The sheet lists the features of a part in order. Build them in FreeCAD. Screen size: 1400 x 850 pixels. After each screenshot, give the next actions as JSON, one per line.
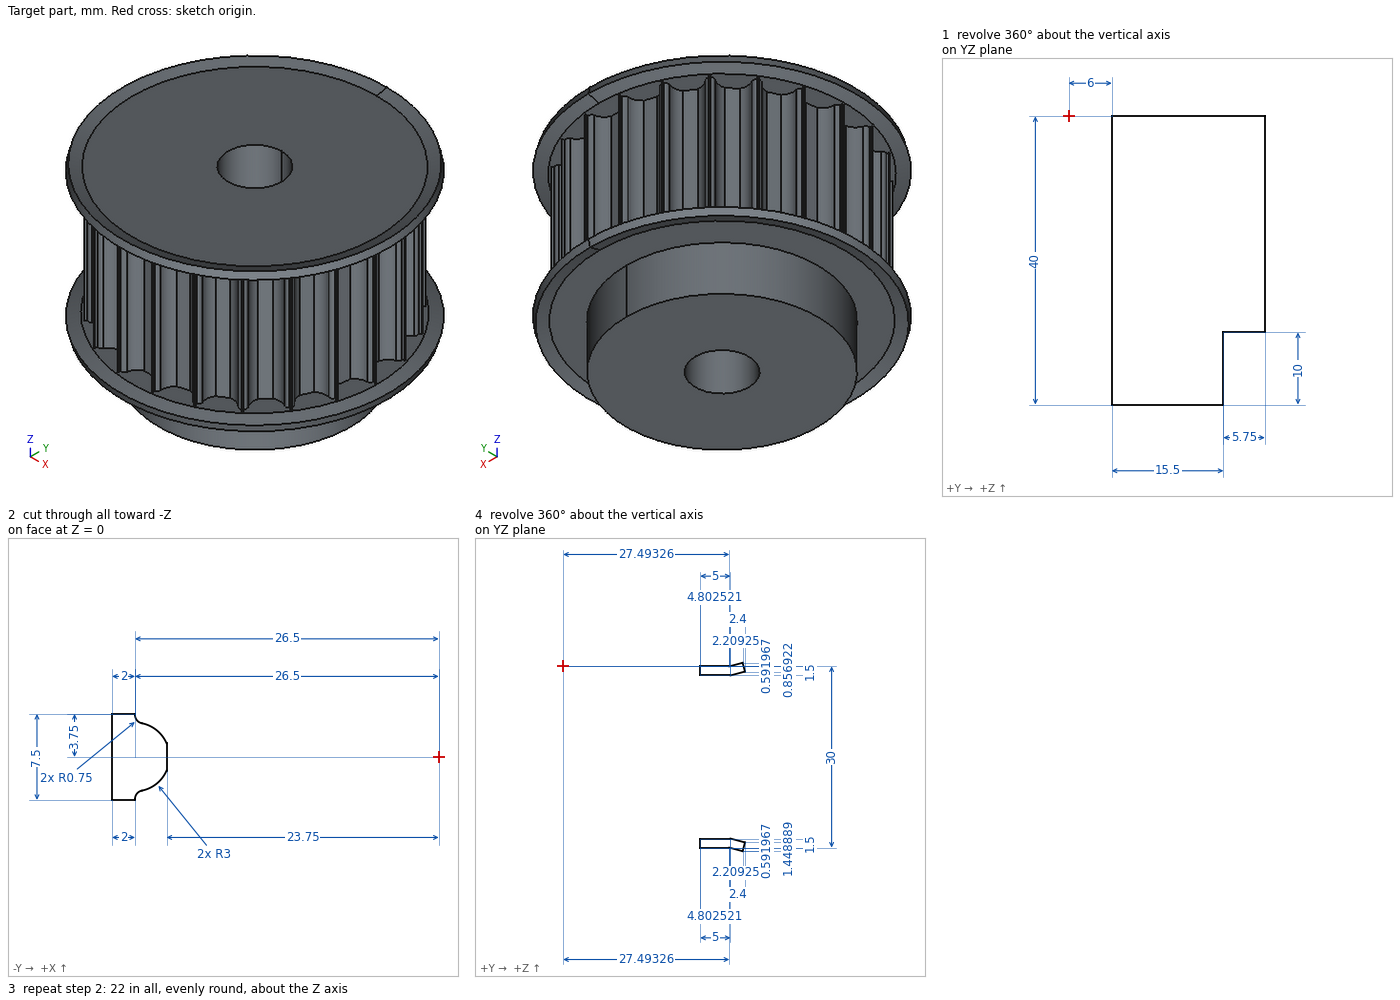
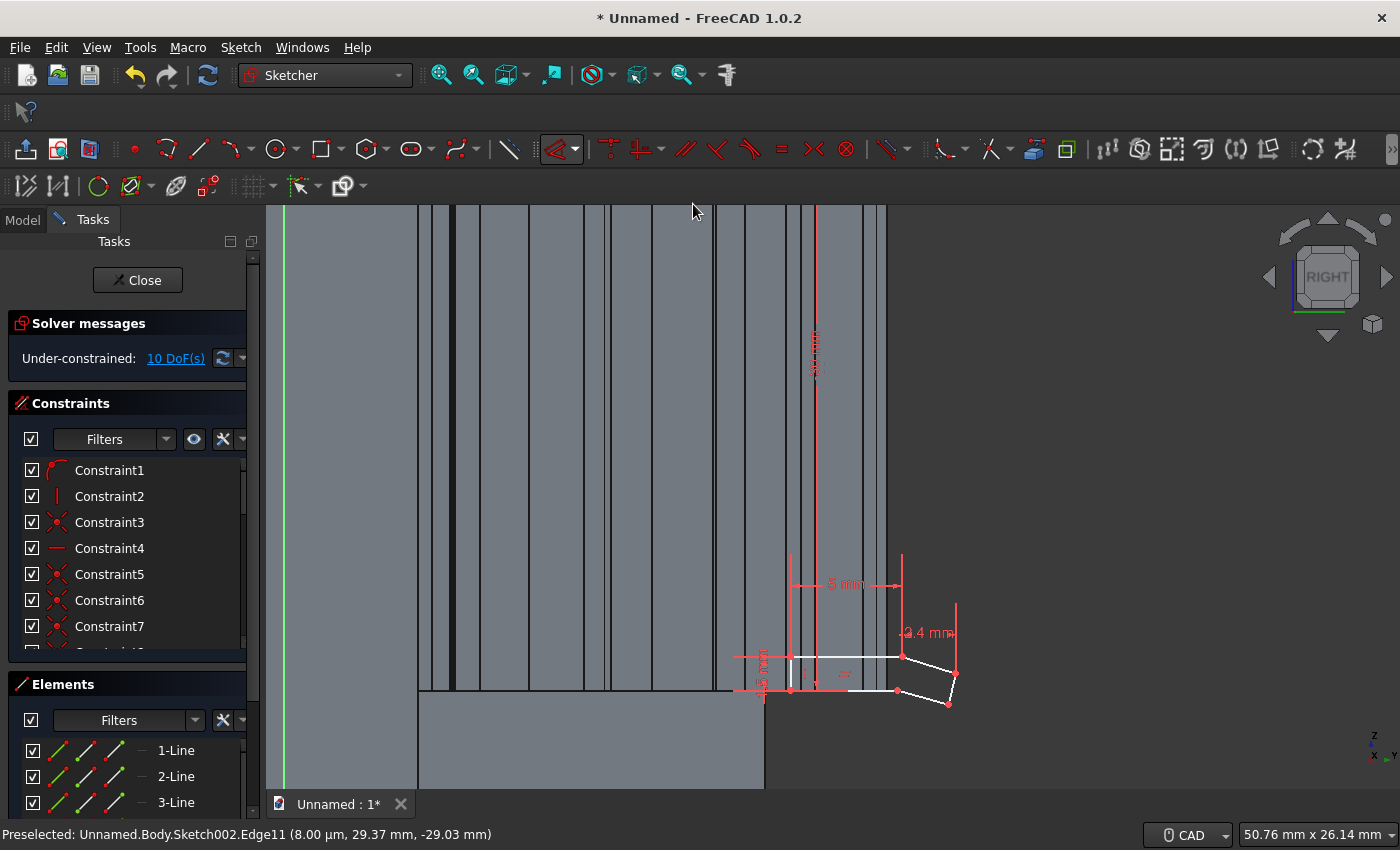
{"action": "scroll", "coordinate": [940, 669], "scroll_direction": "down", "scroll_amount": 3}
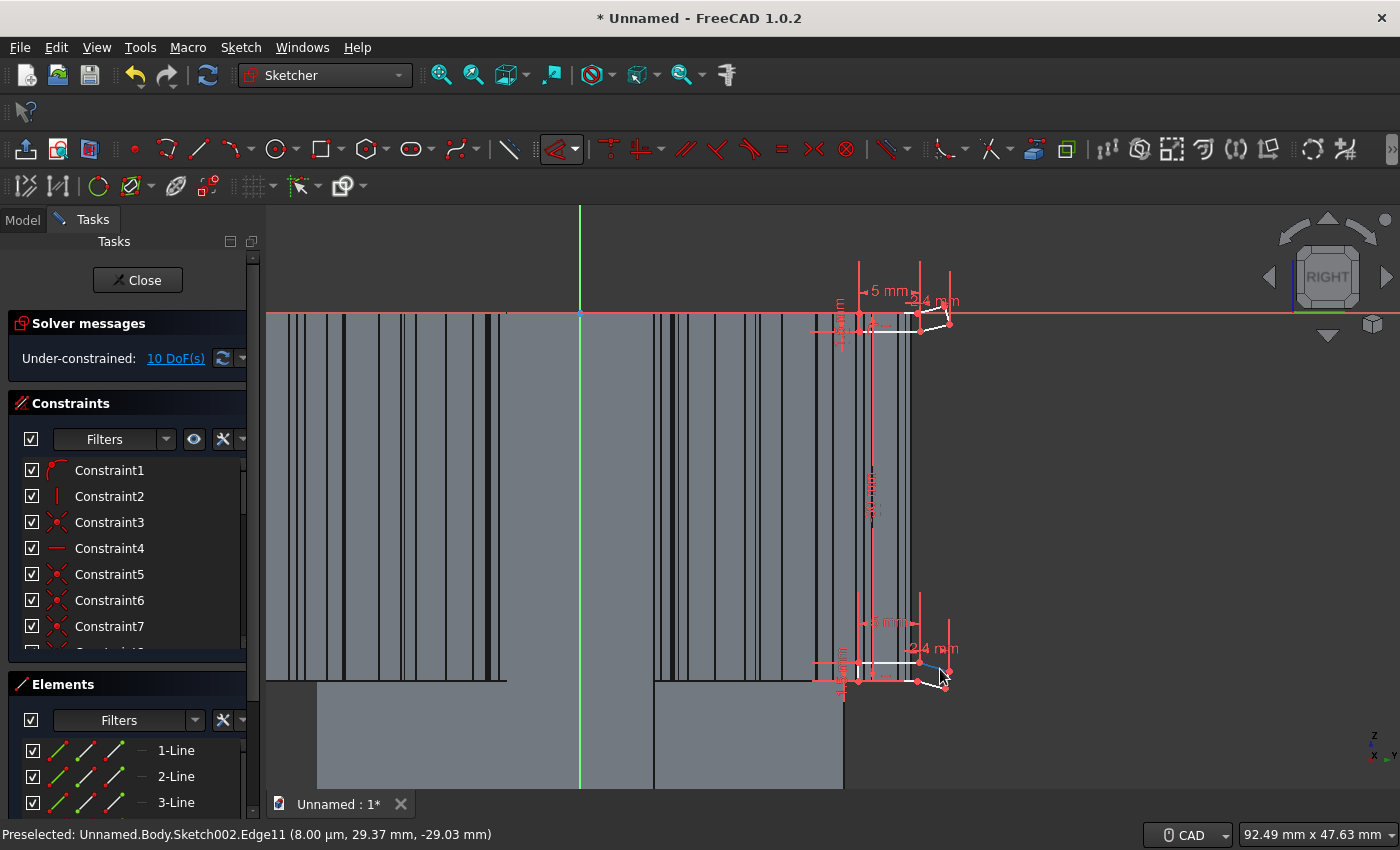
{"action": "left_click", "coordinate": [900, 313]}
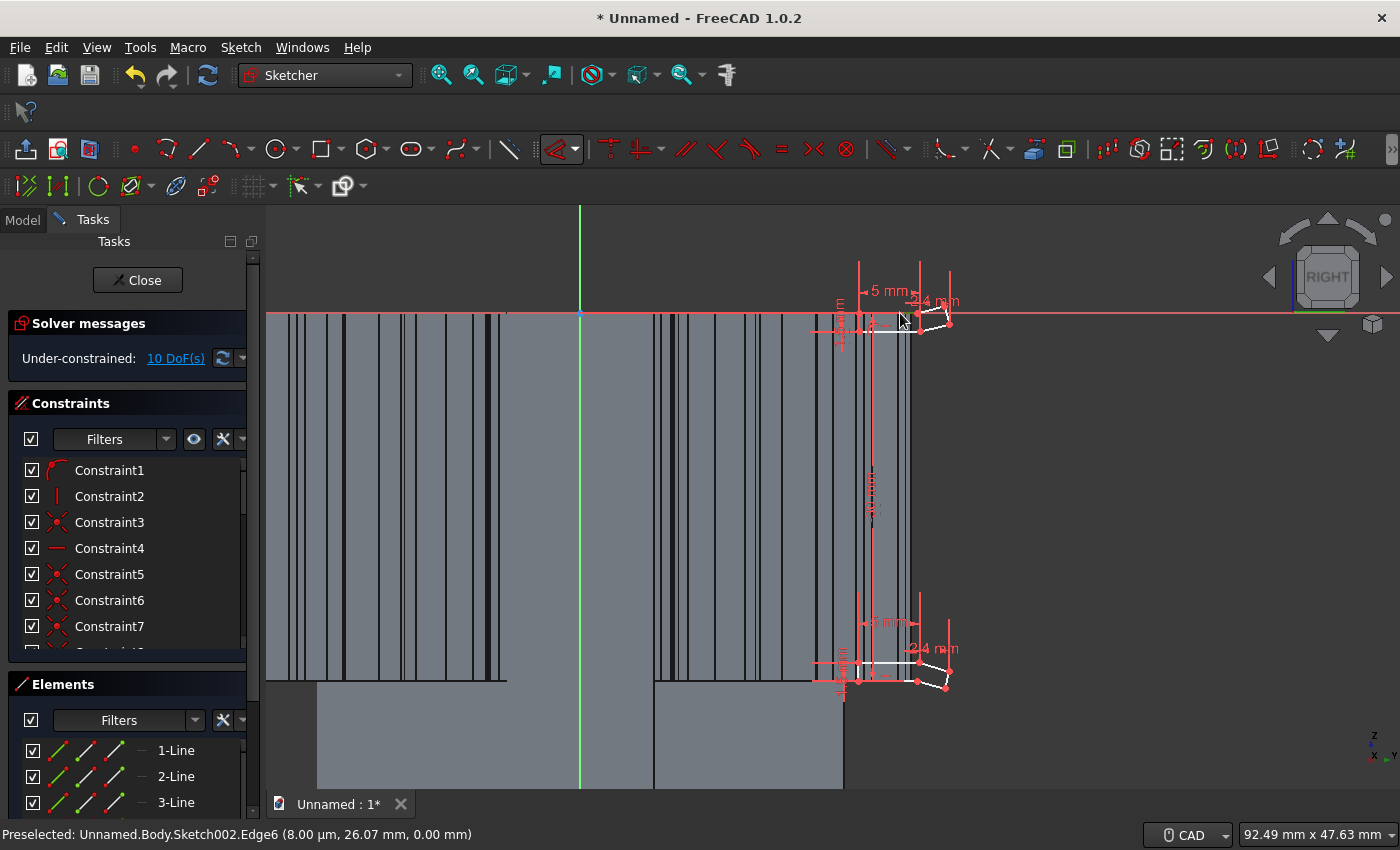
{"action": "left_click", "coordinate": [578, 150]}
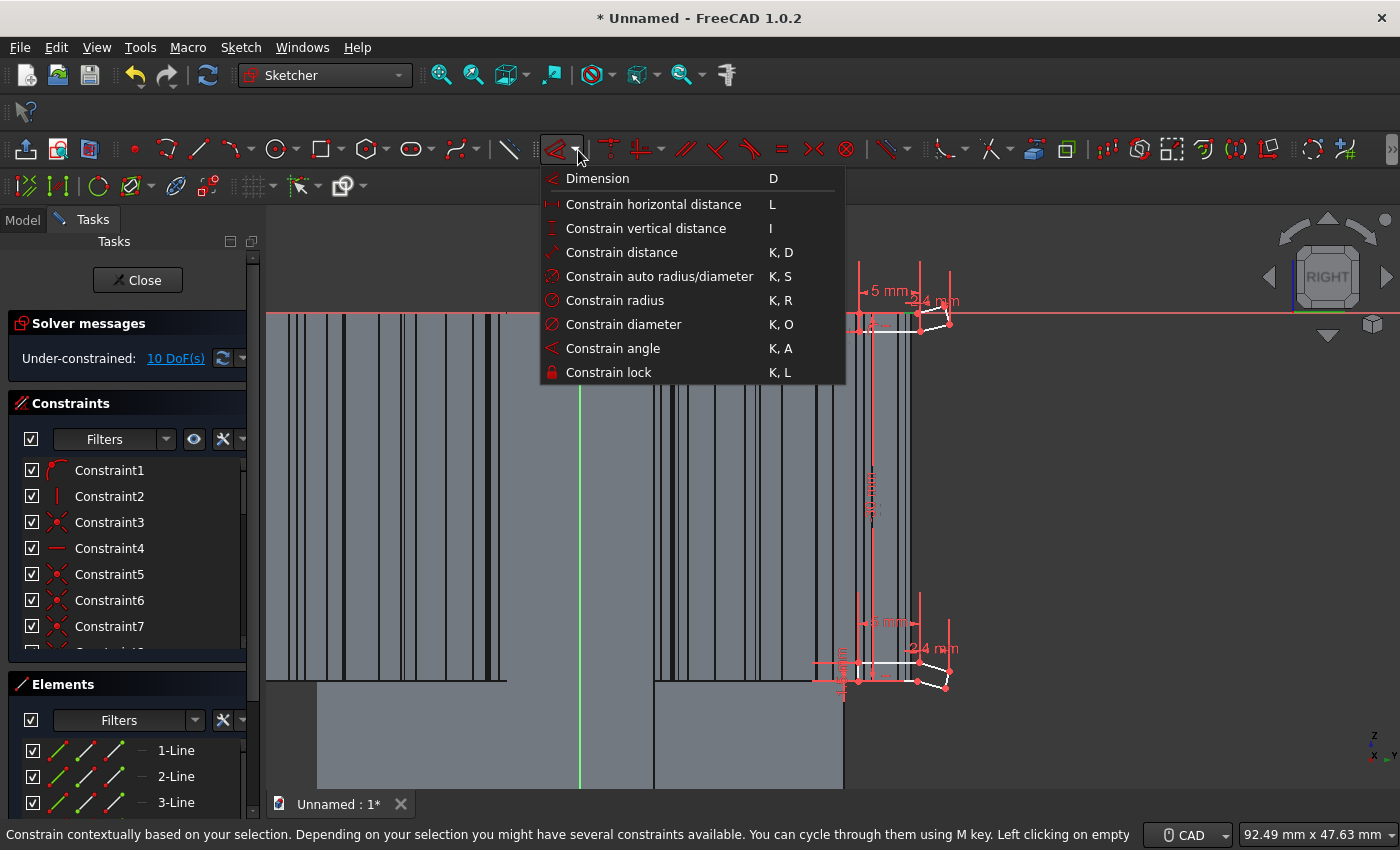
{"action": "left_click", "coordinate": [693, 204]}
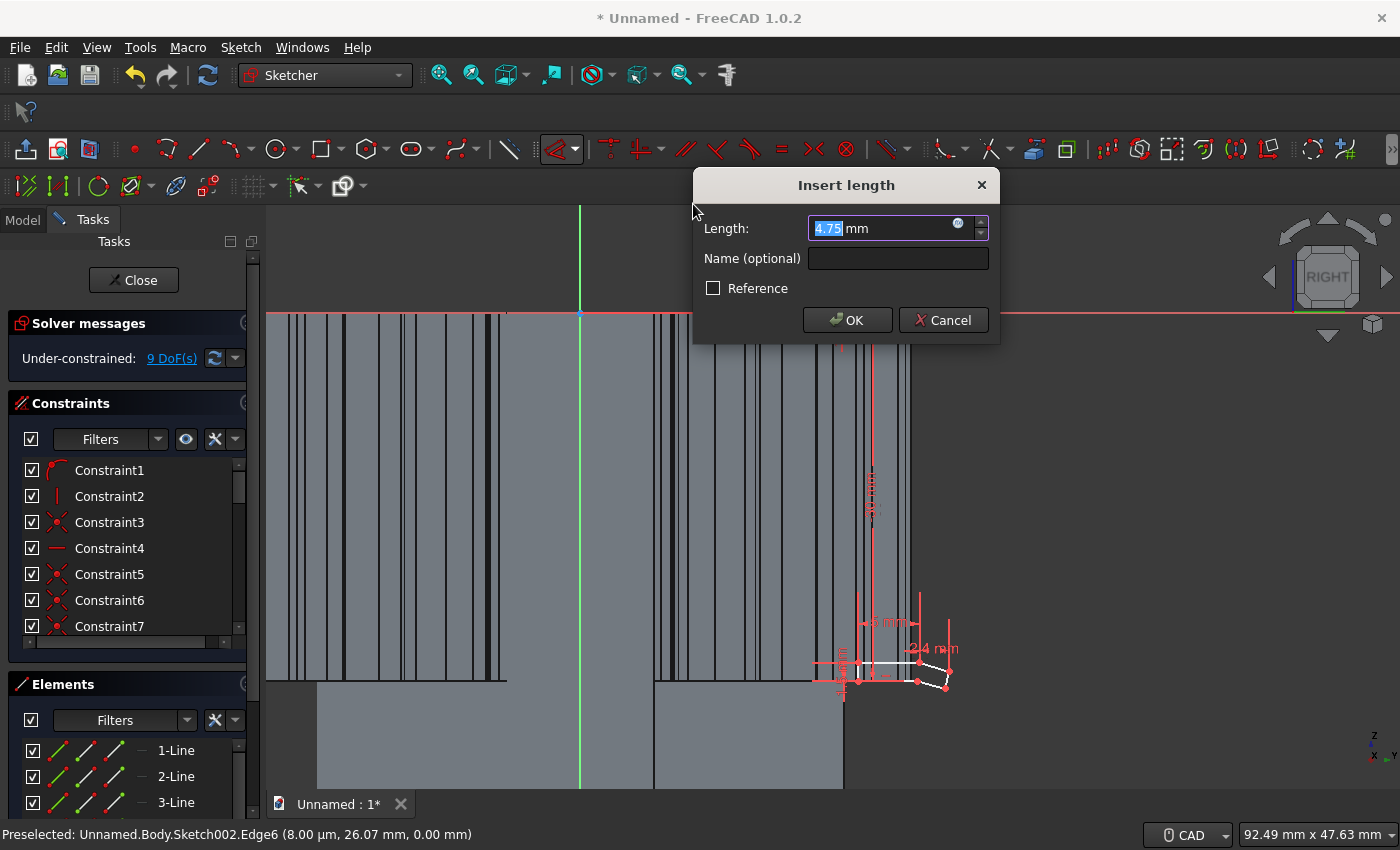
{"action": "type", "text": "4.802521"}
{"action": "key", "text": "Return"}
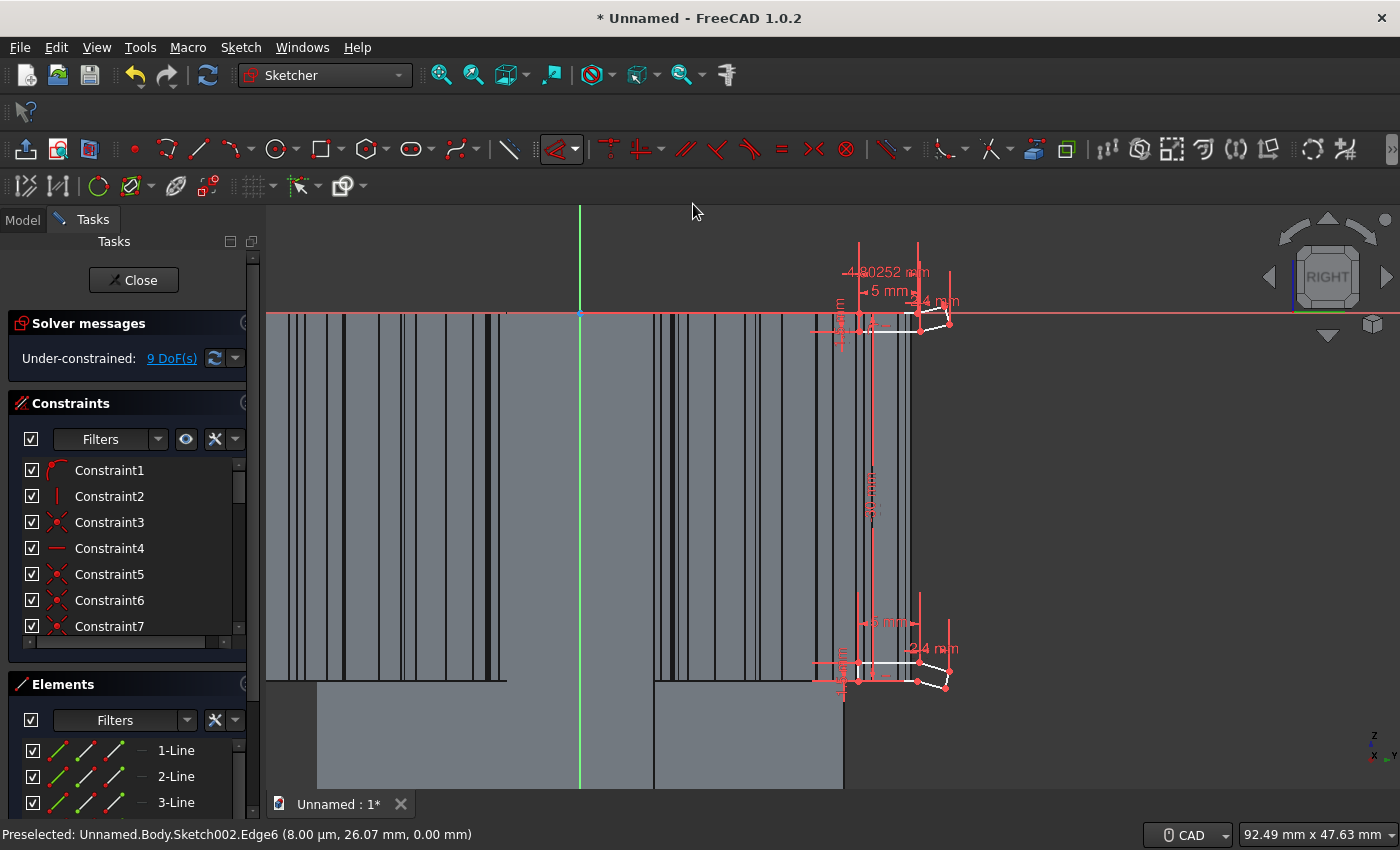
{"action": "left_click", "coordinate": [876, 681]}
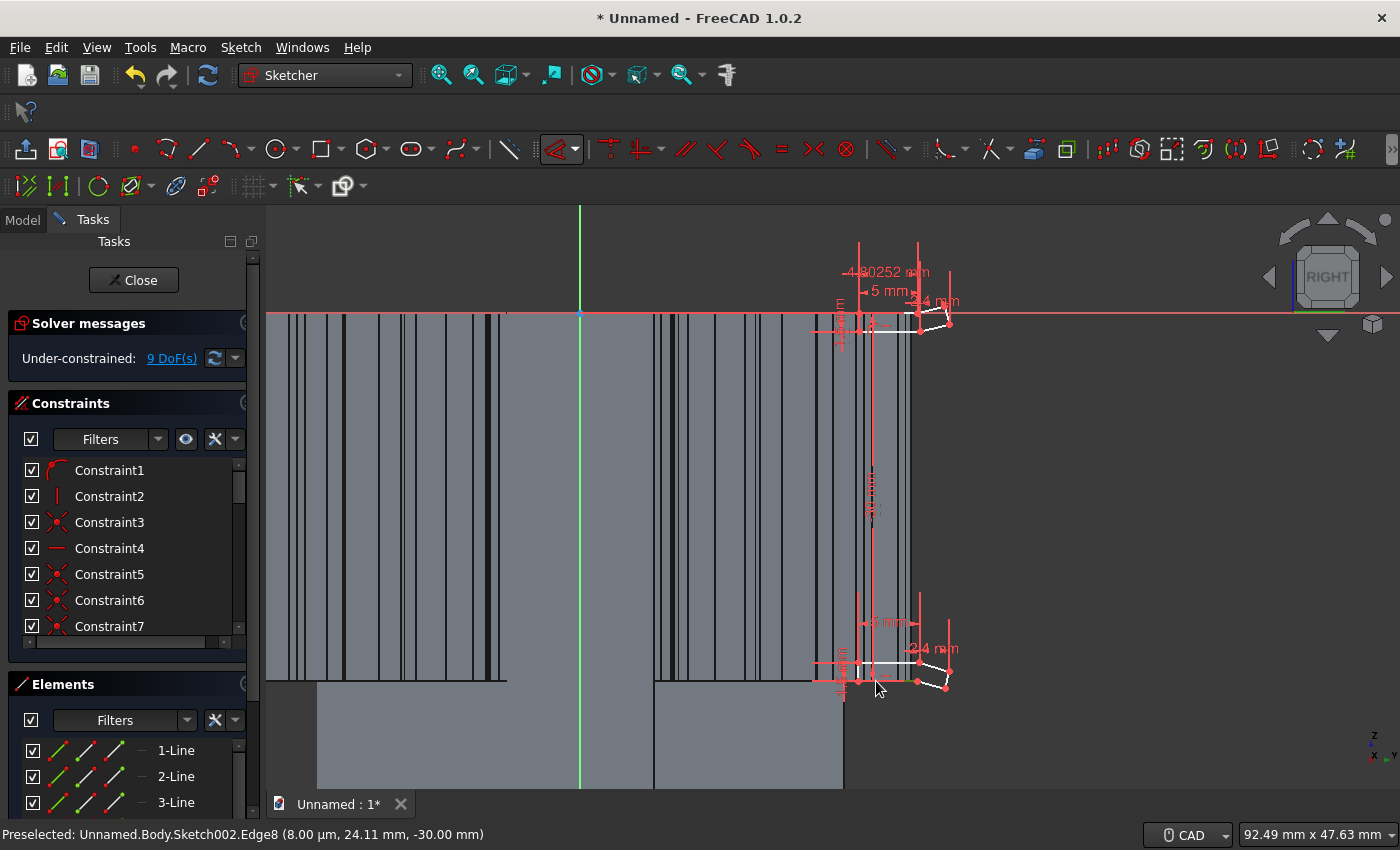
{"action": "key", "text": "l"}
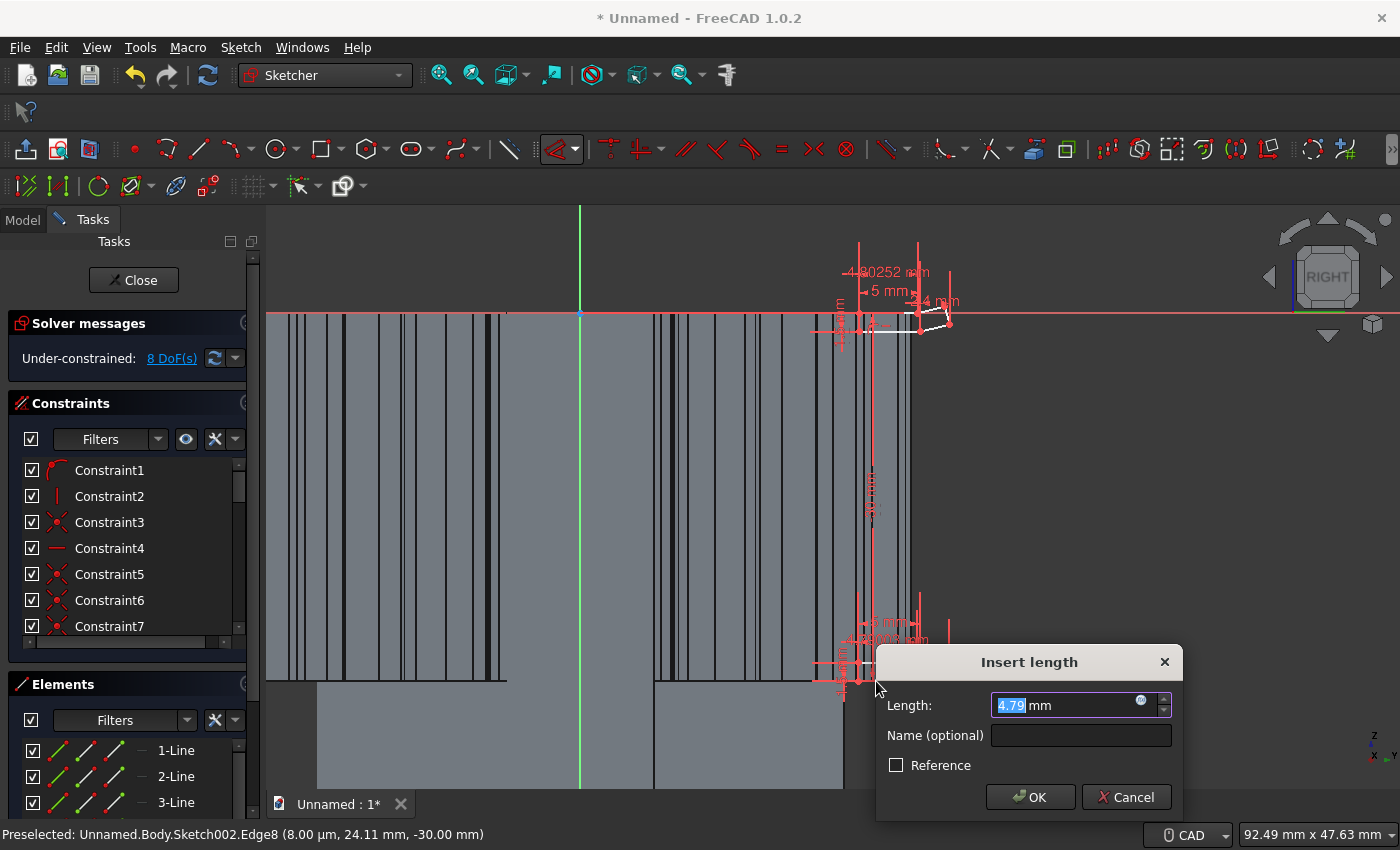
{"action": "type", "text": "4.802521"}
{"action": "key", "text": "Return"}